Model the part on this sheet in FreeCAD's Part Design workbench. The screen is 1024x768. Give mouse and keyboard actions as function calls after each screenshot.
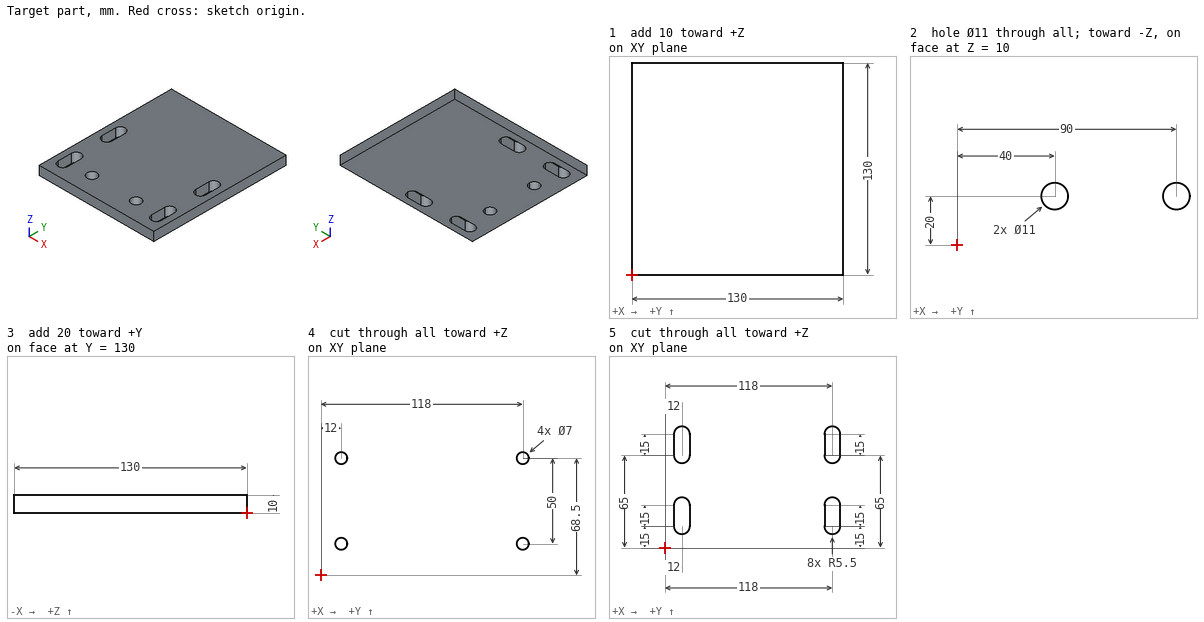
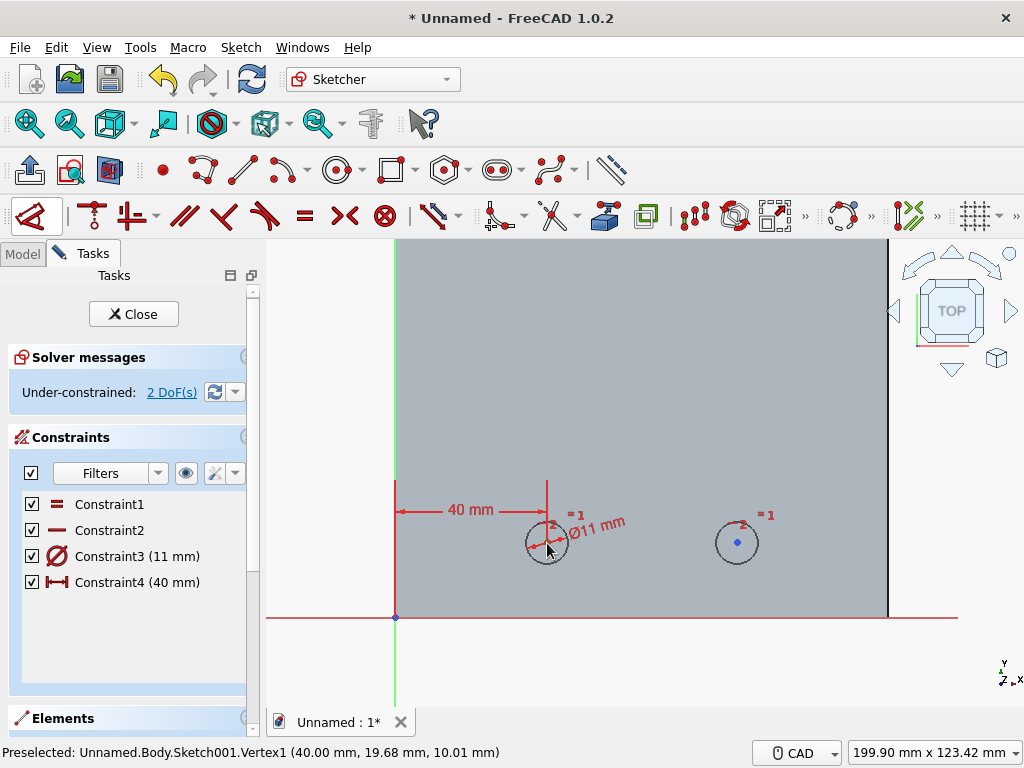
key(i)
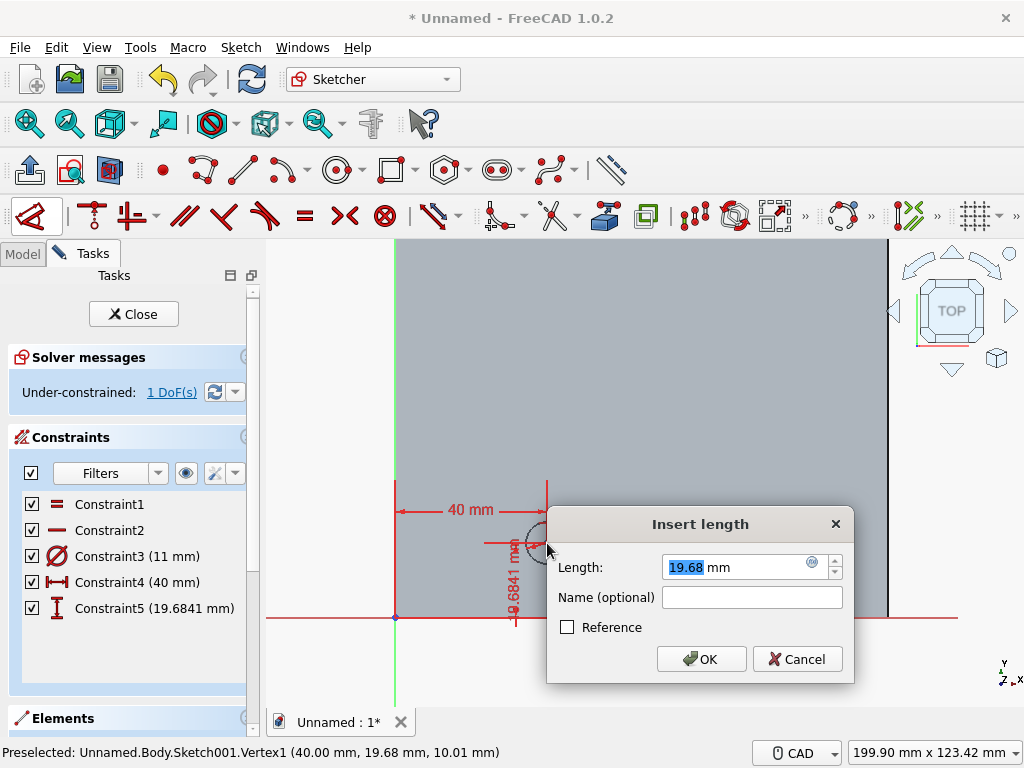
text(20)
key(Return)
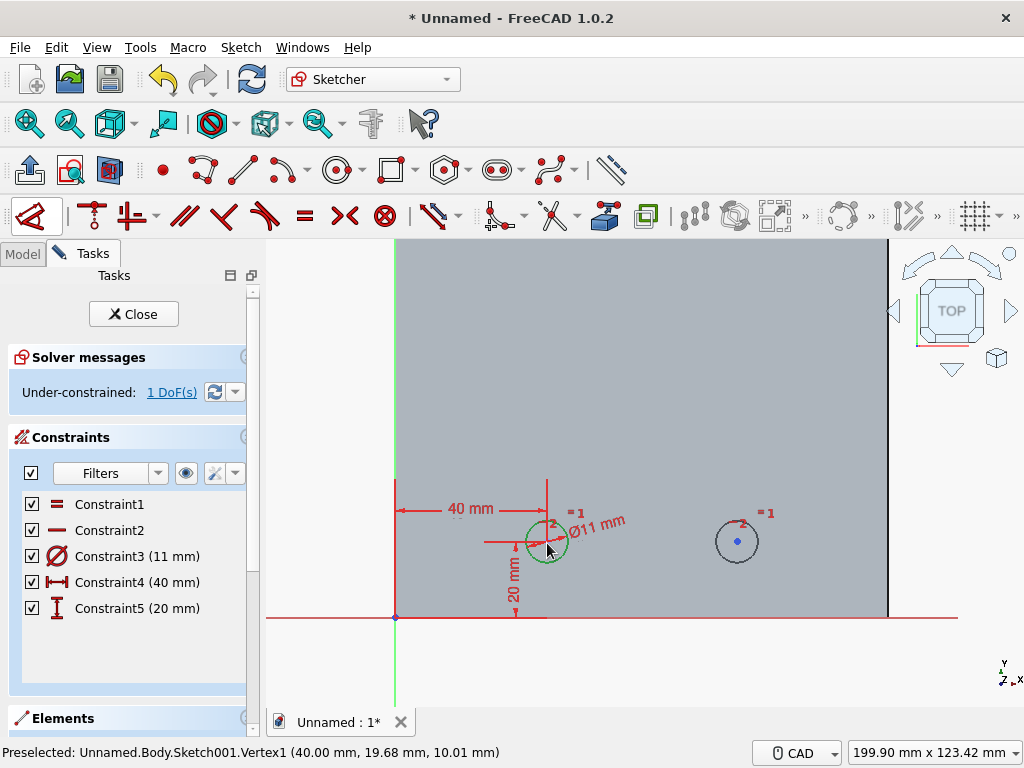
click(737, 542)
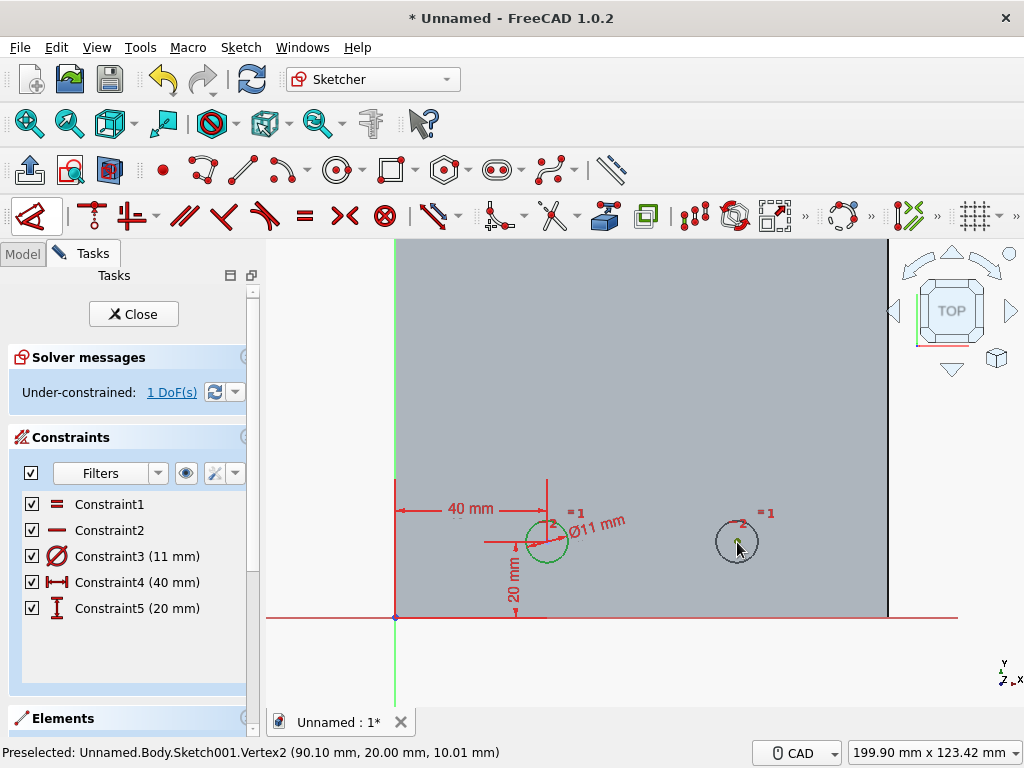
click(56, 216)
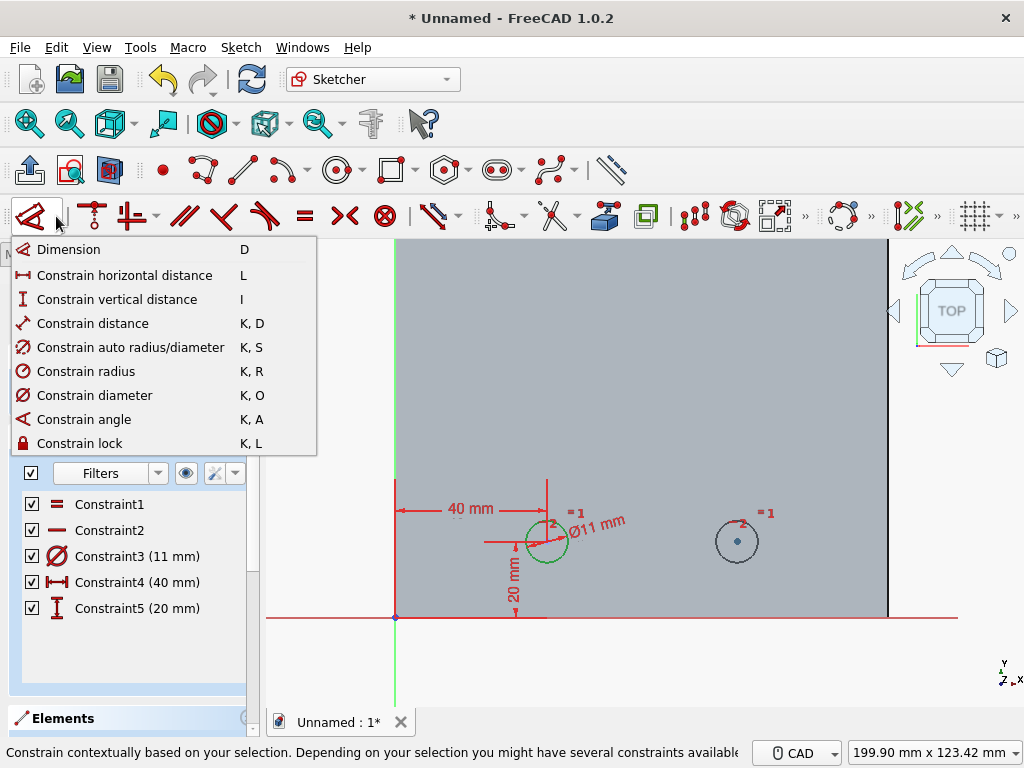
click(164, 275)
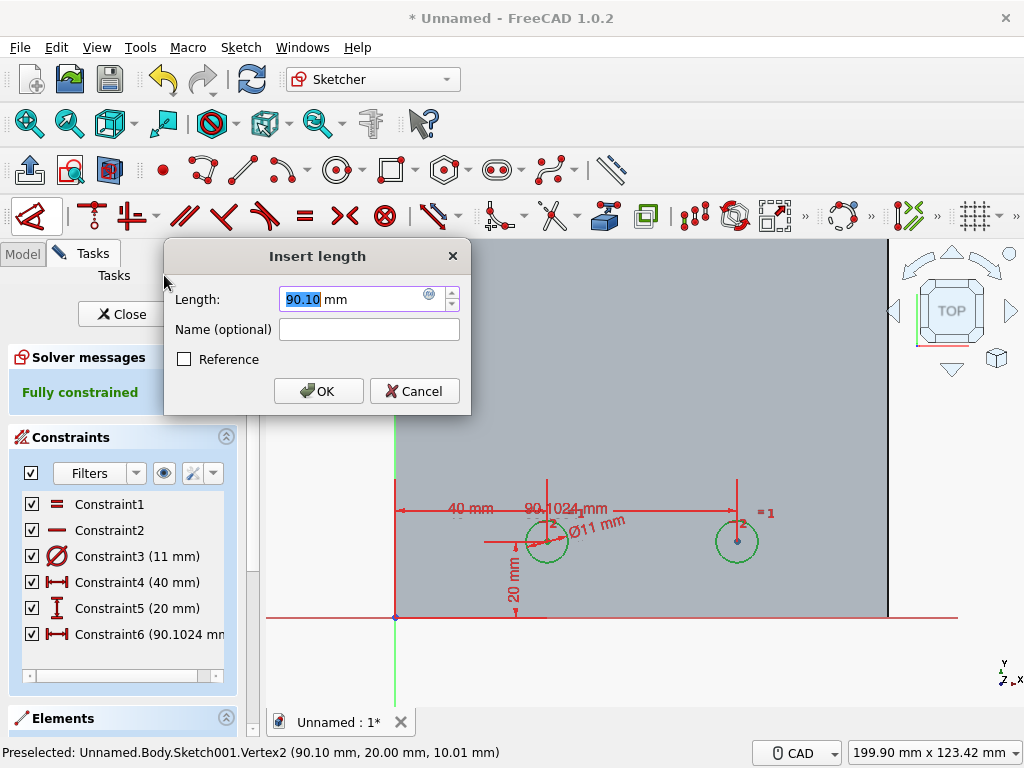
text(90)
key(Return)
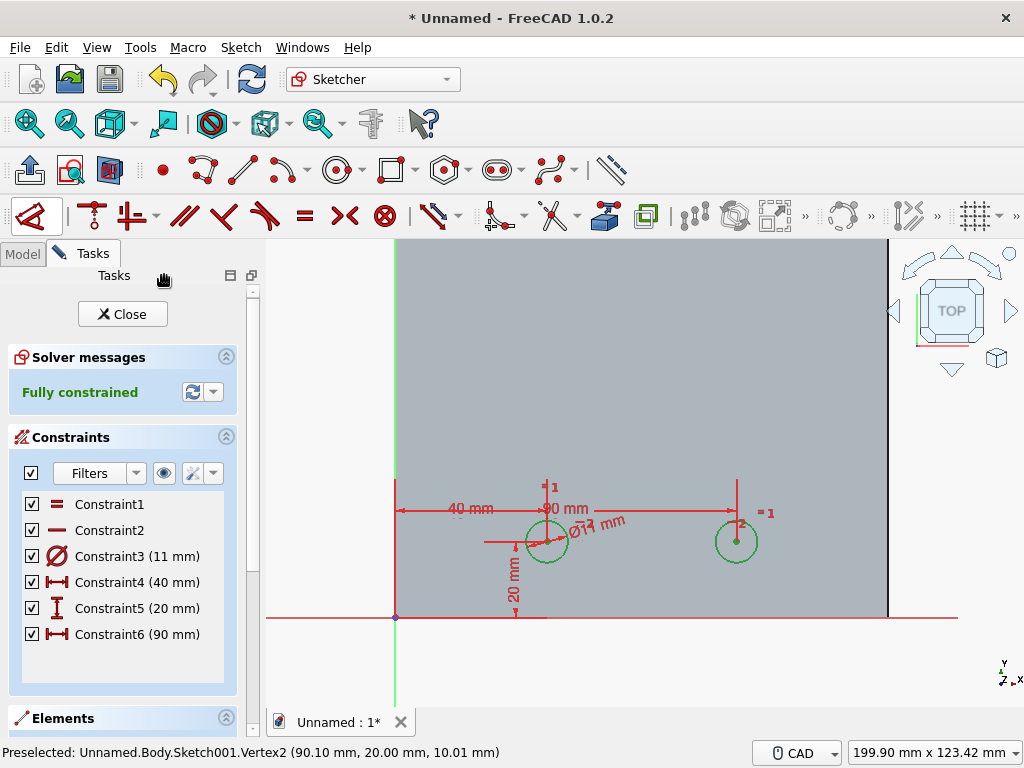
click(123, 314)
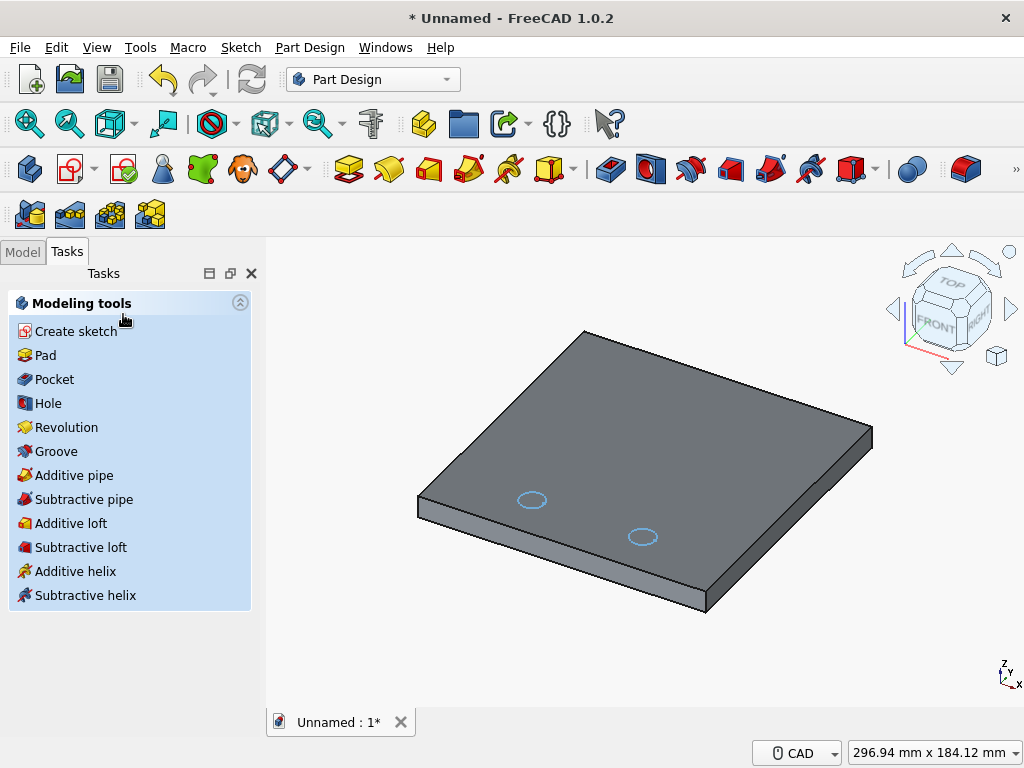
click(652, 170)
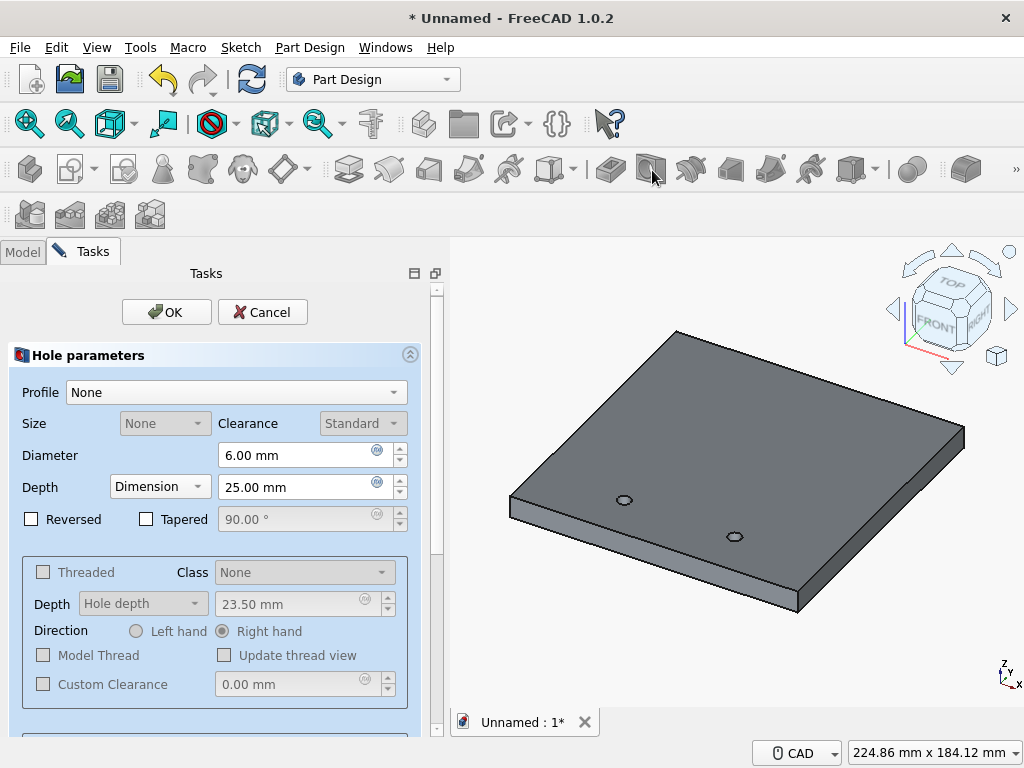
triple_click(305, 455)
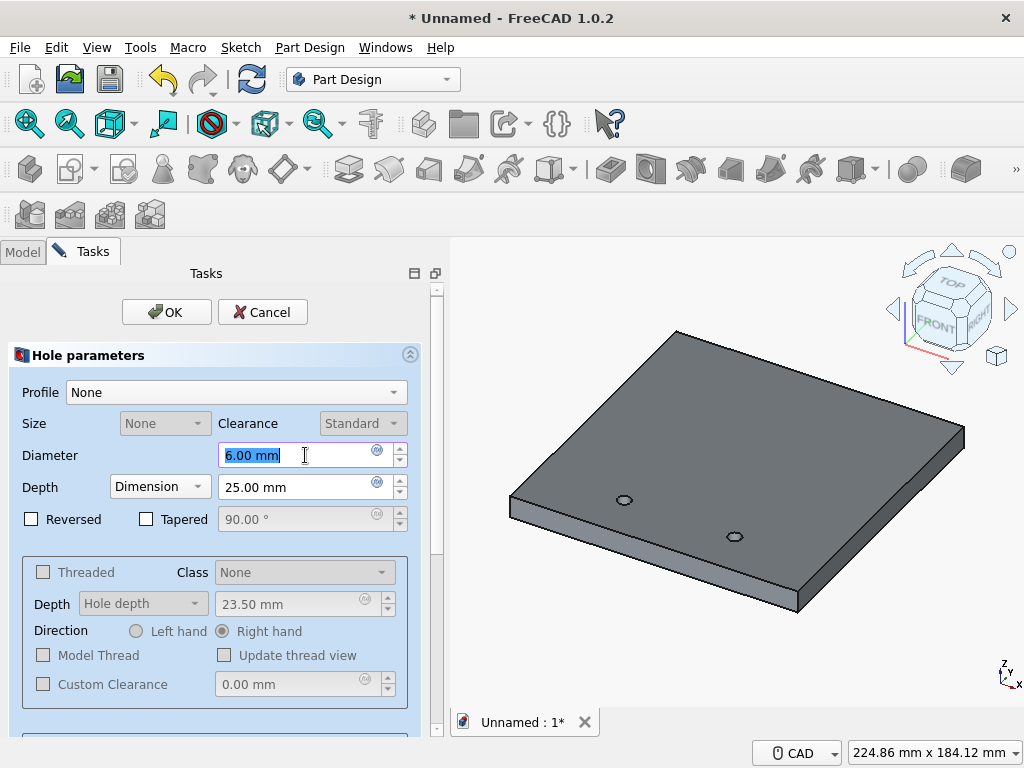
text(11)
key(Tab)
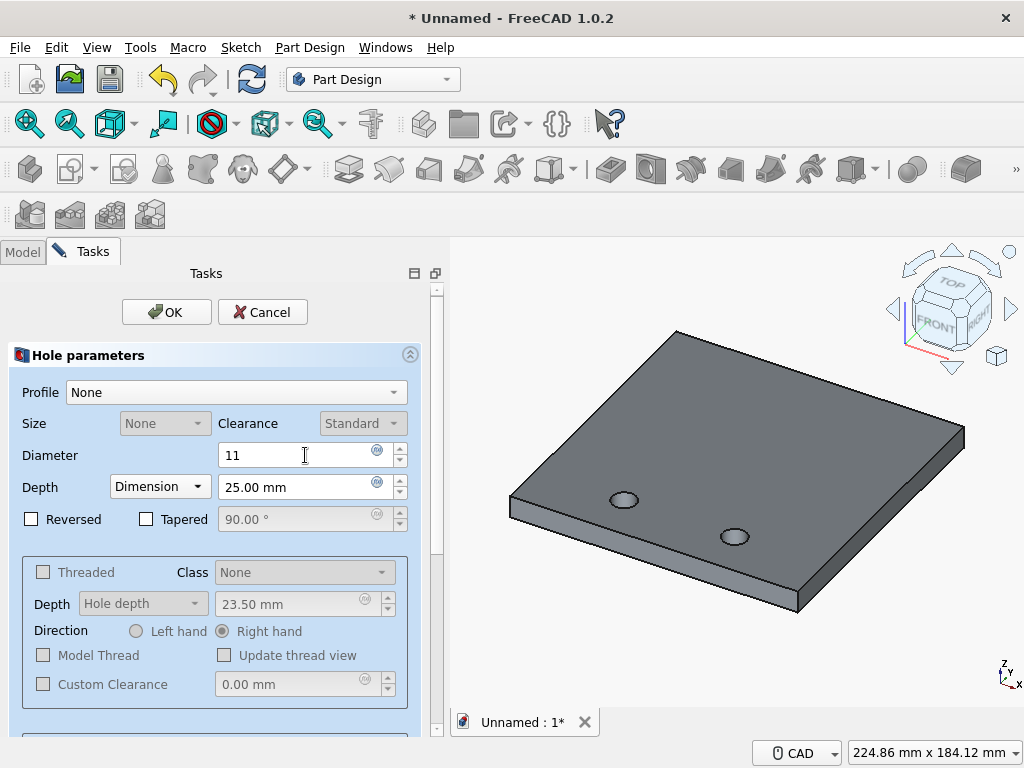
click(161, 486)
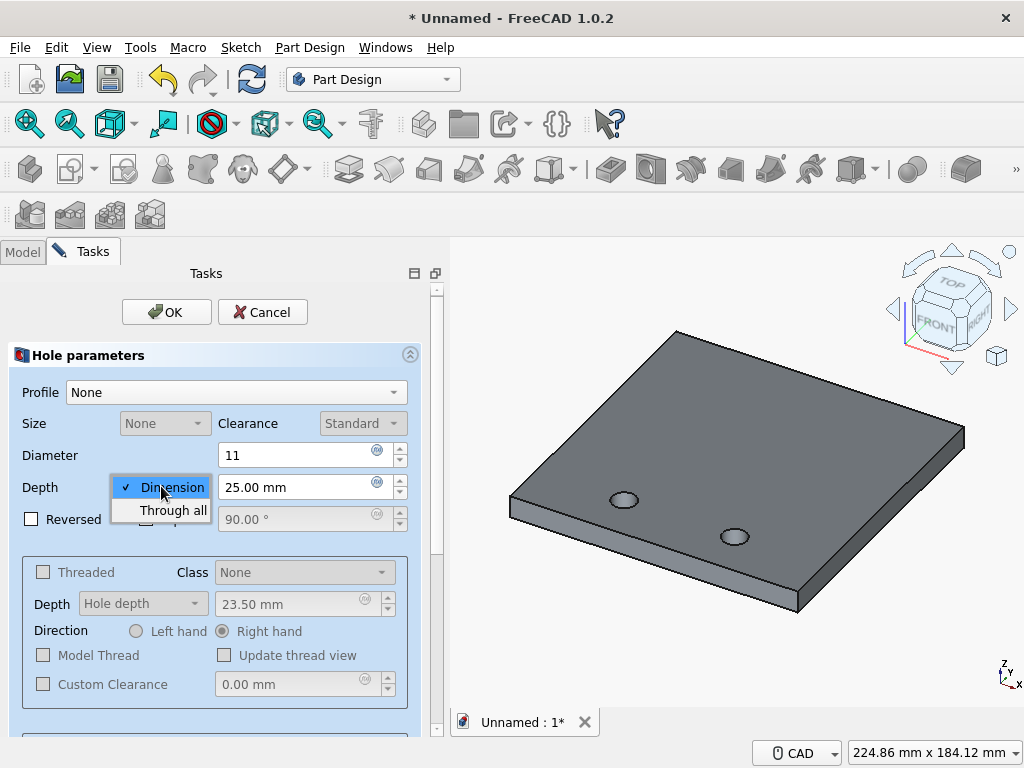
click(160, 510)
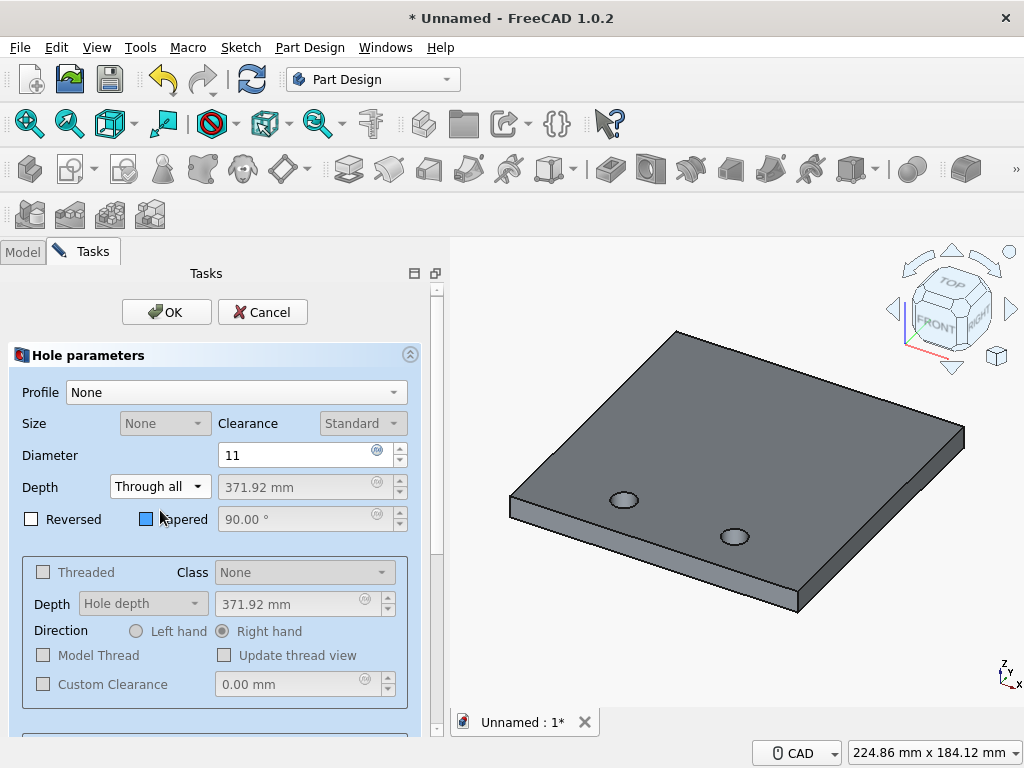
click(167, 312)